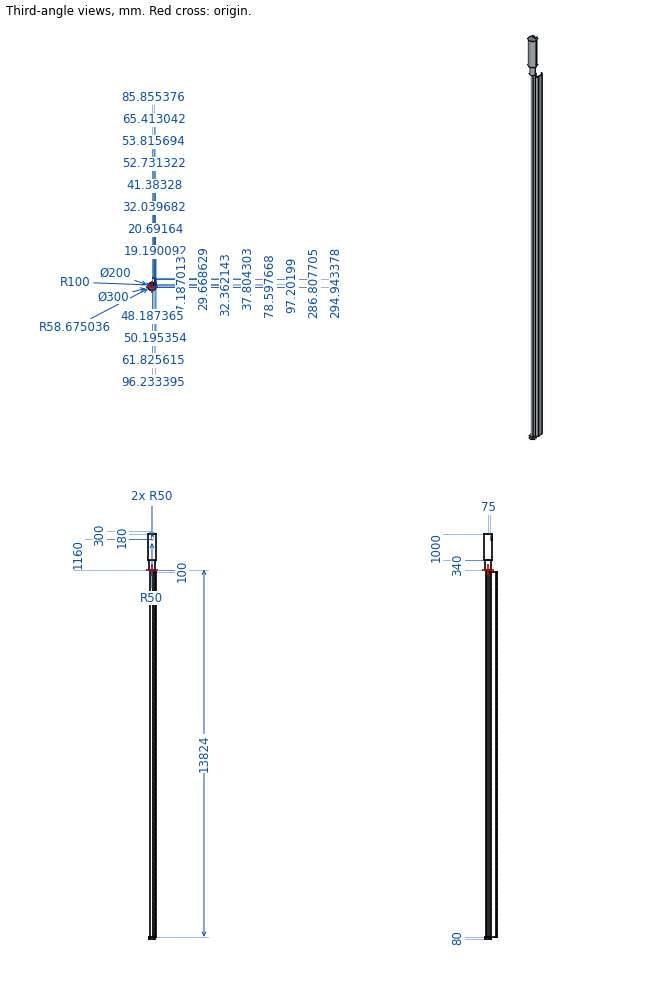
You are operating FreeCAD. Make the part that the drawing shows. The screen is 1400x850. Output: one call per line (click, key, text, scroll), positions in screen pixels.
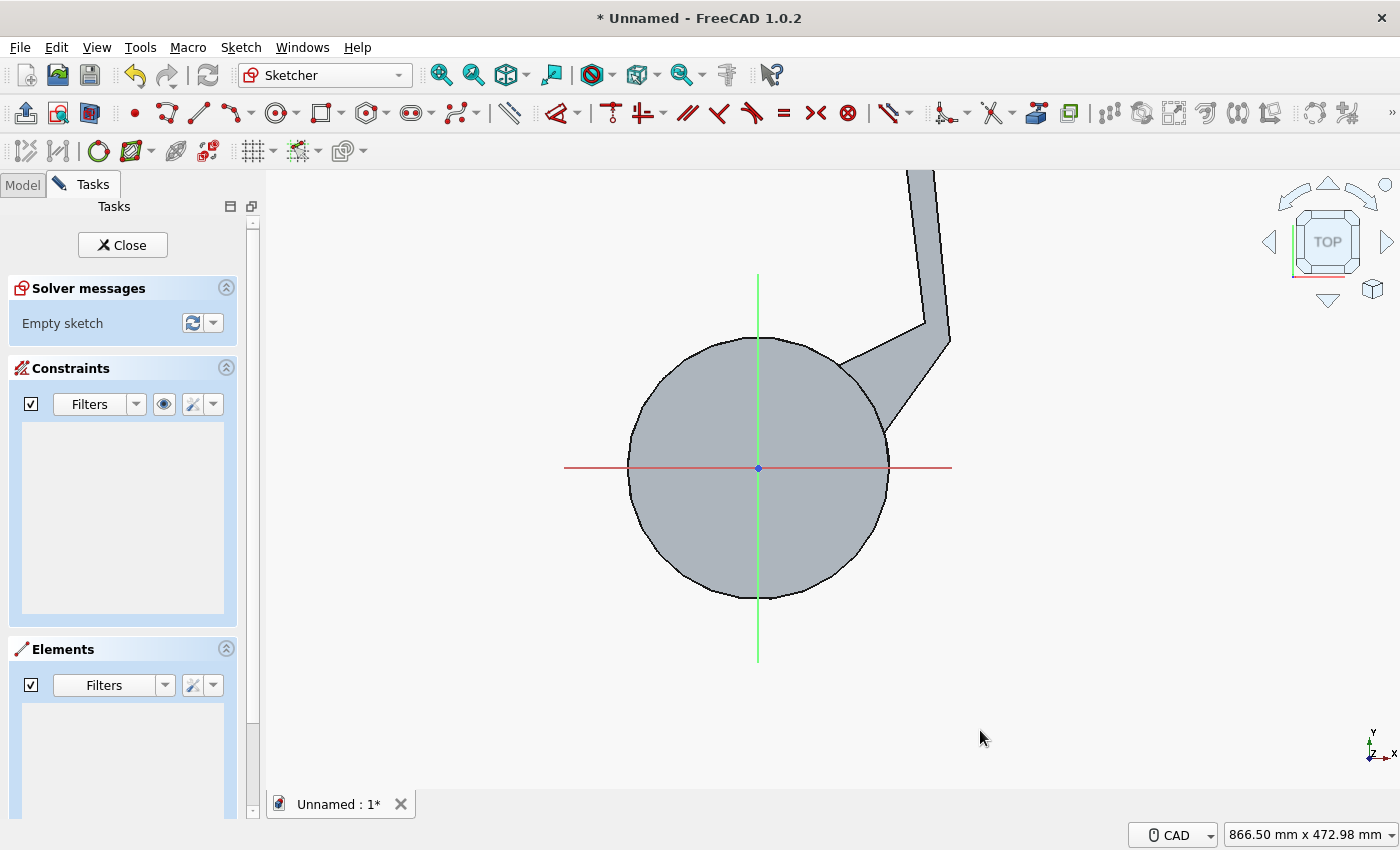
key(g)
key(c)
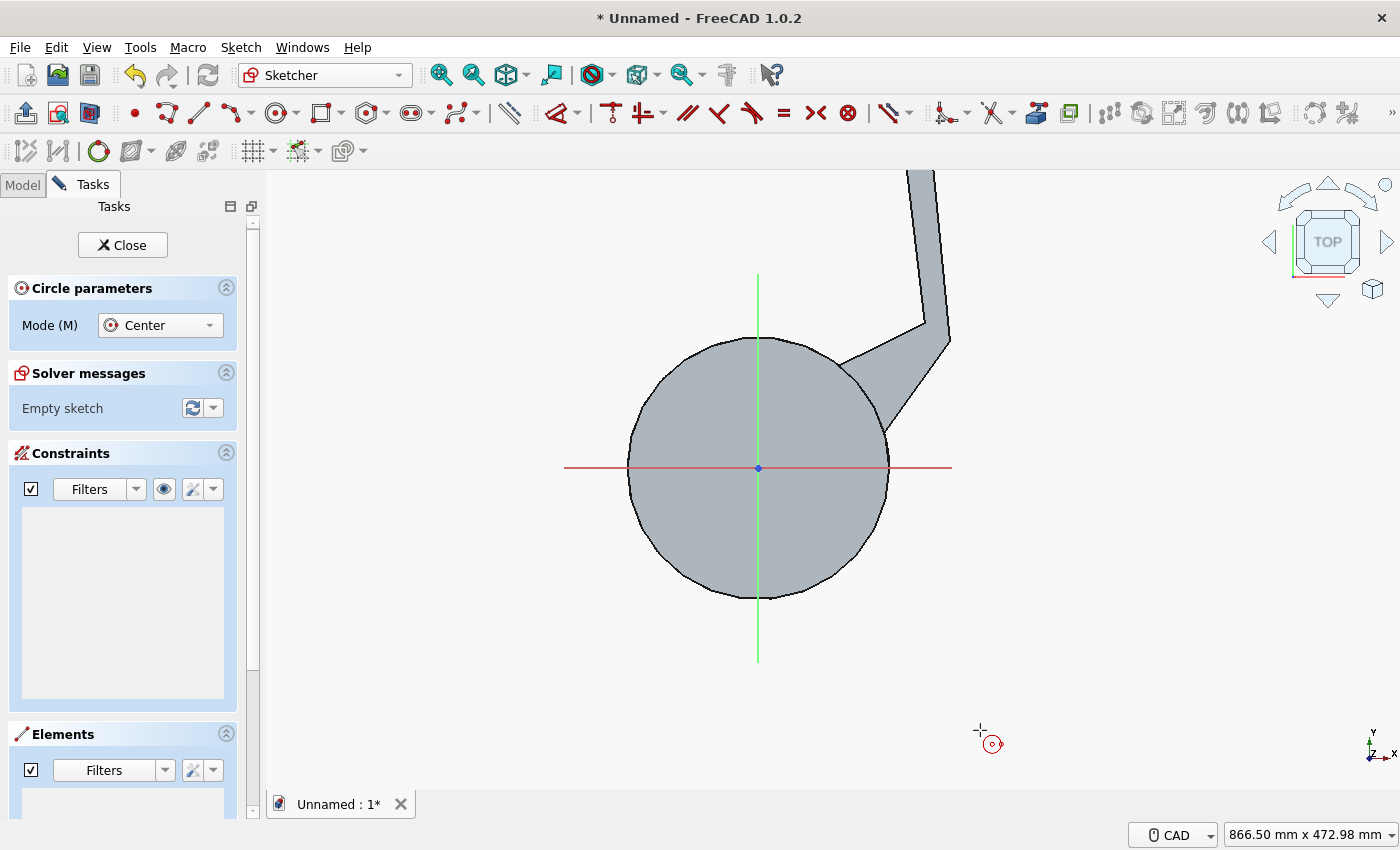
click(758, 468)
click(897, 330)
key(Escape)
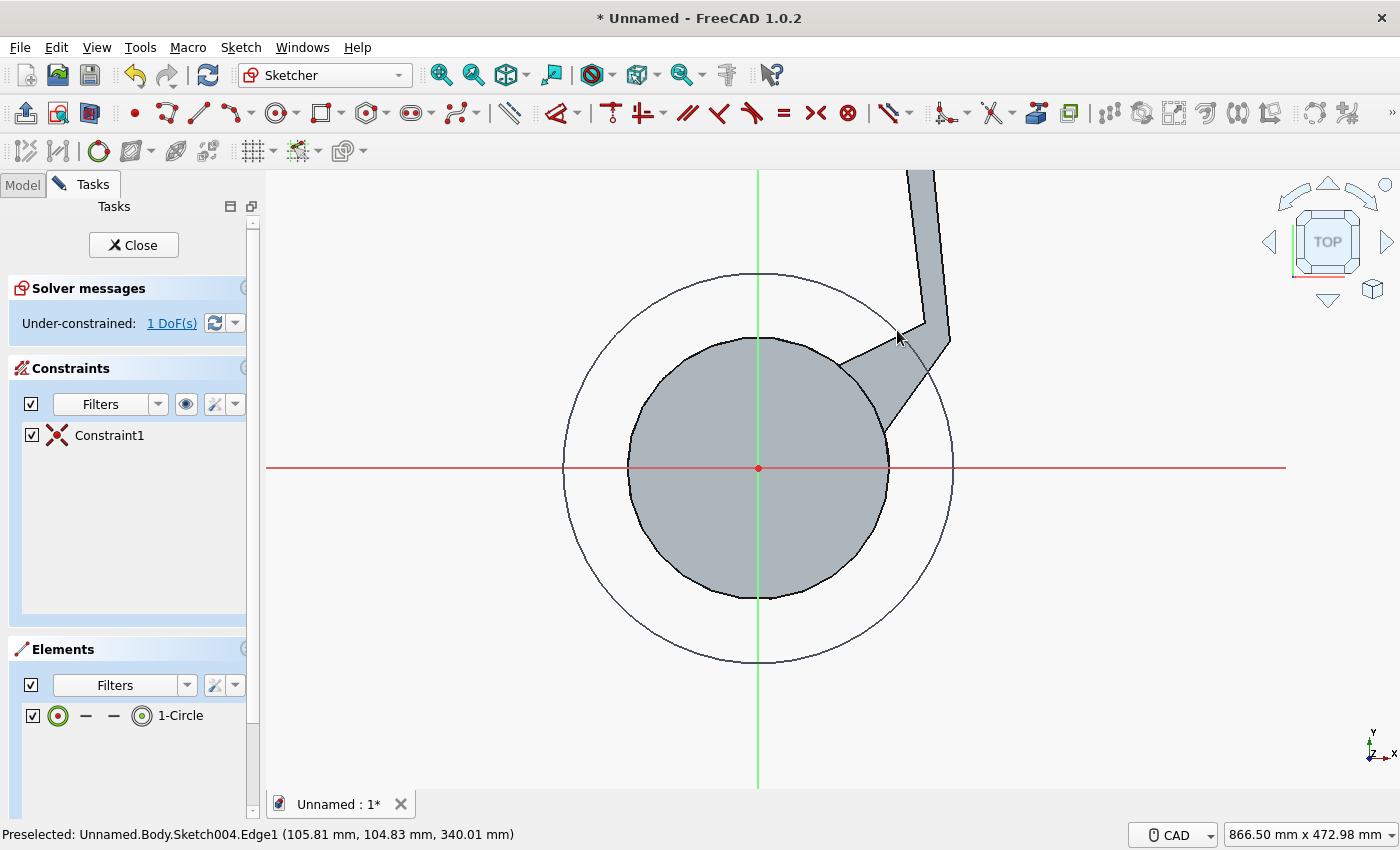
key(d)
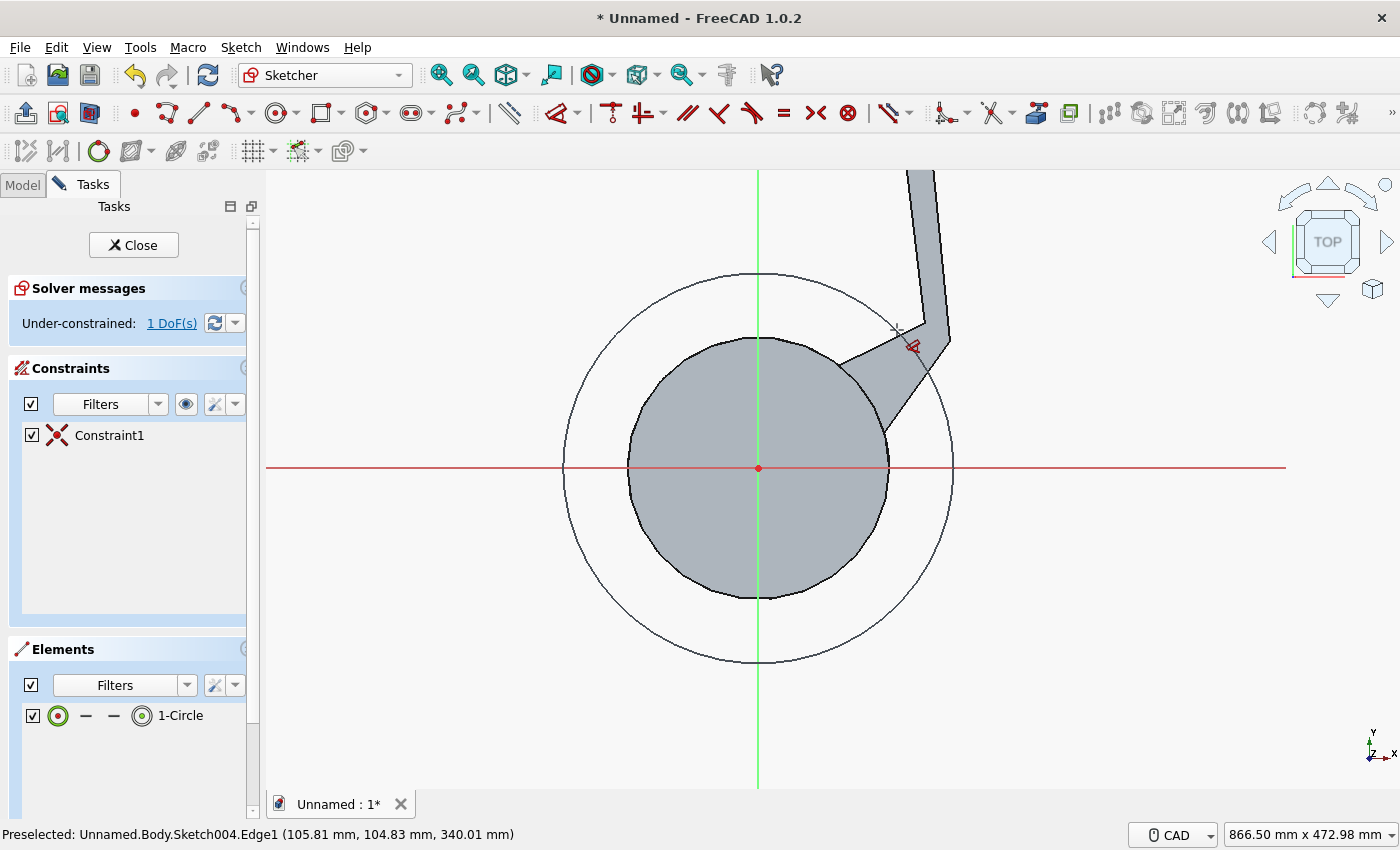
click(896, 330)
click(919, 307)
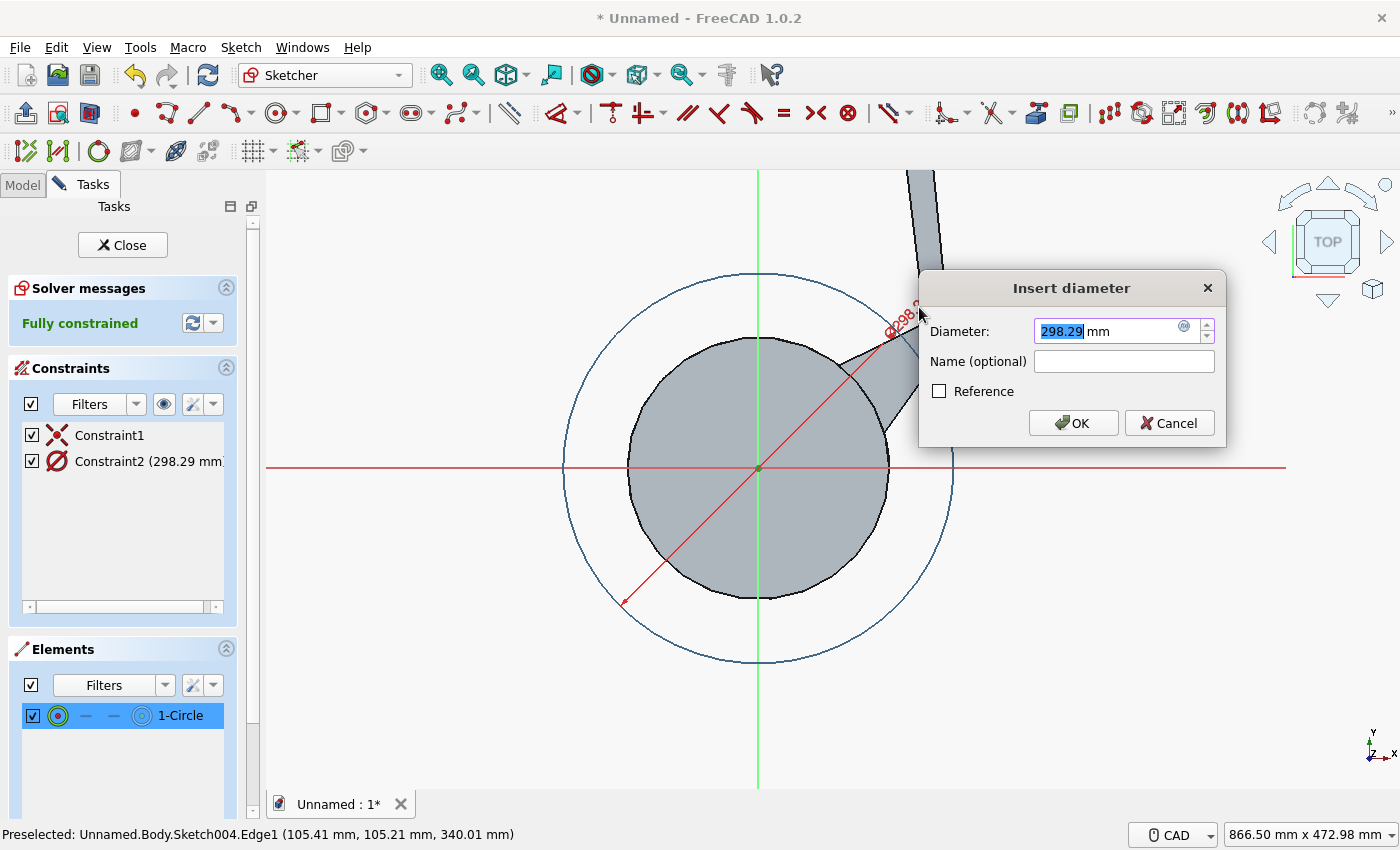
text(300)
key(Return)
key(Escape)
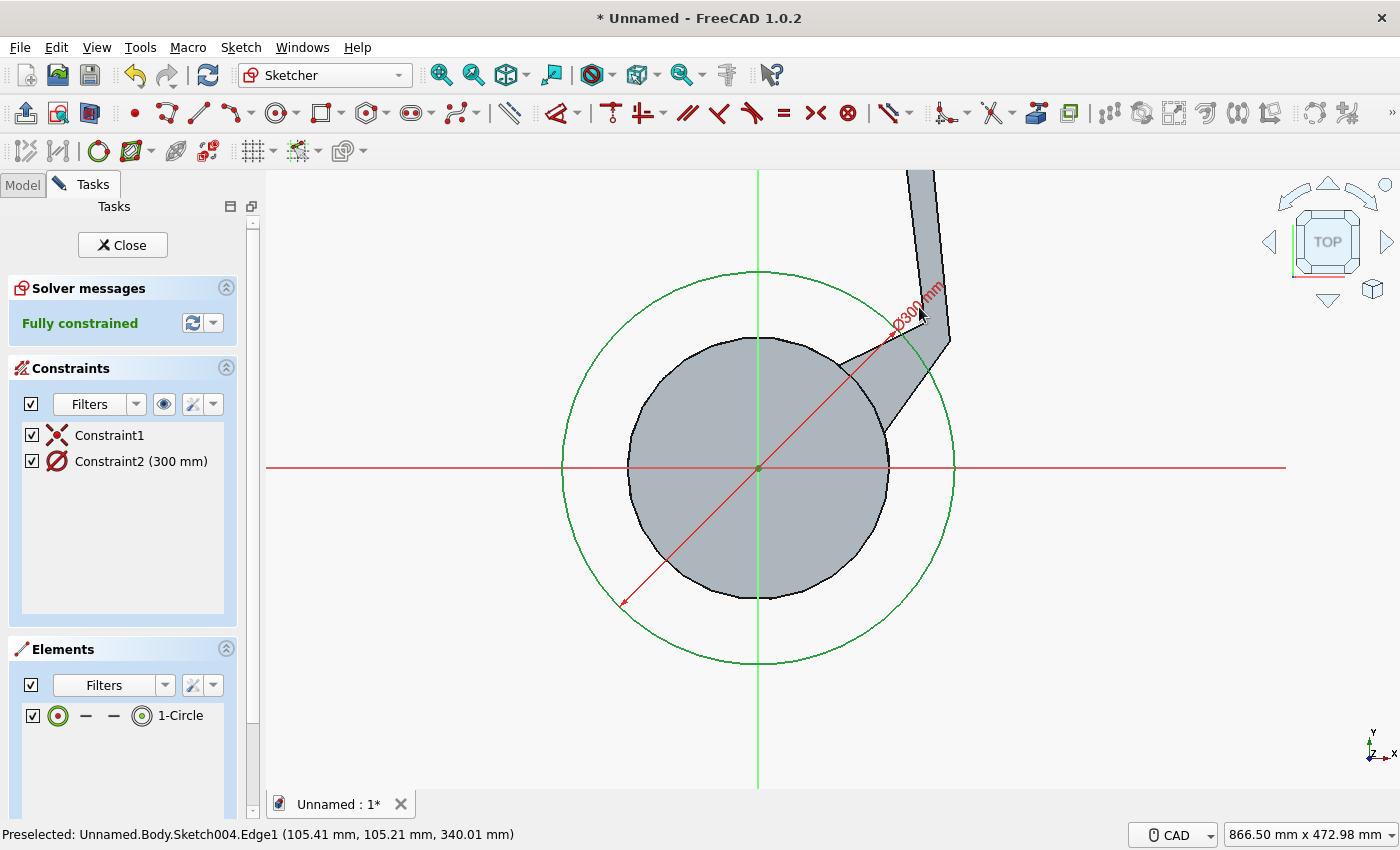
click(123, 245)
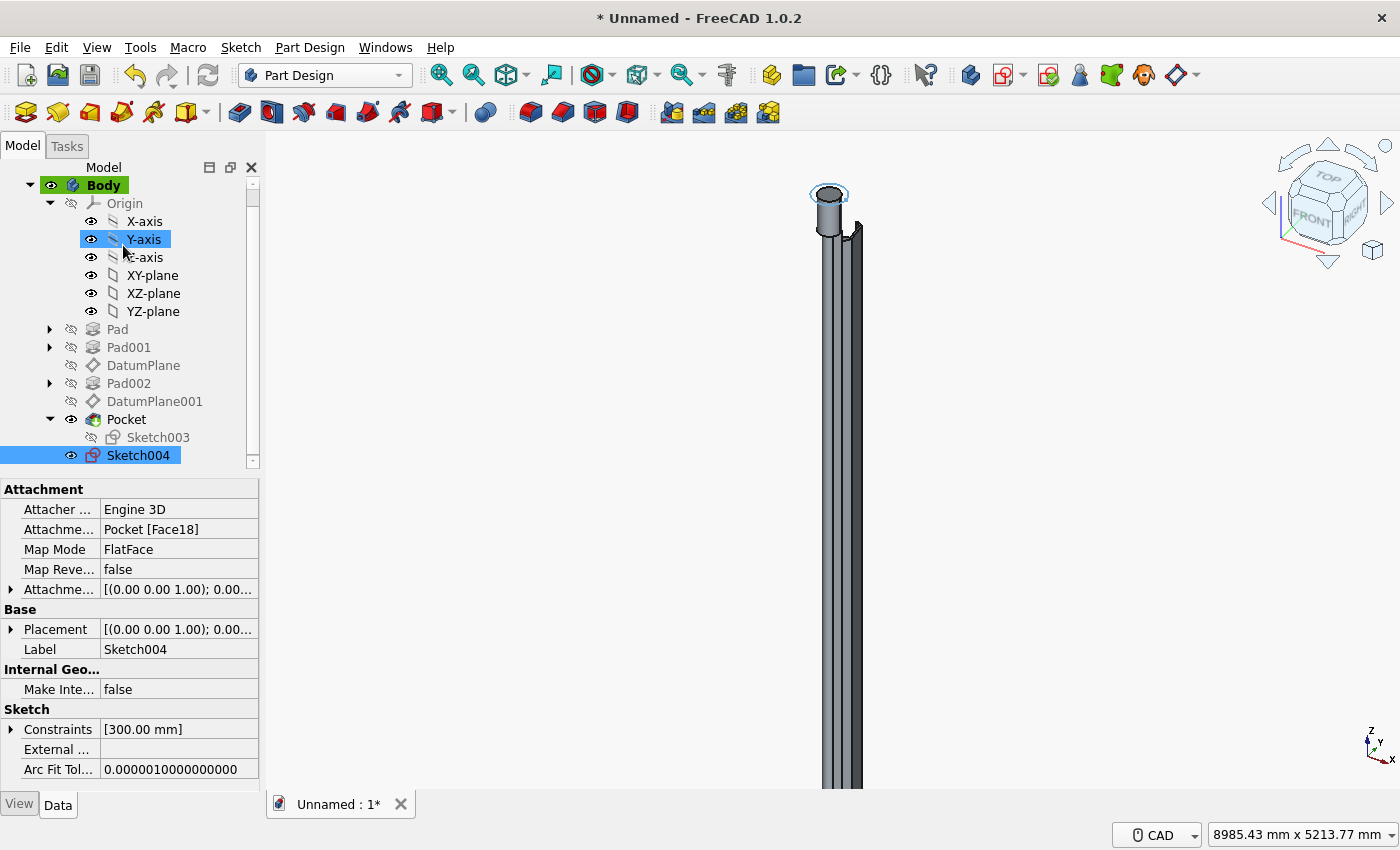
click(26, 112)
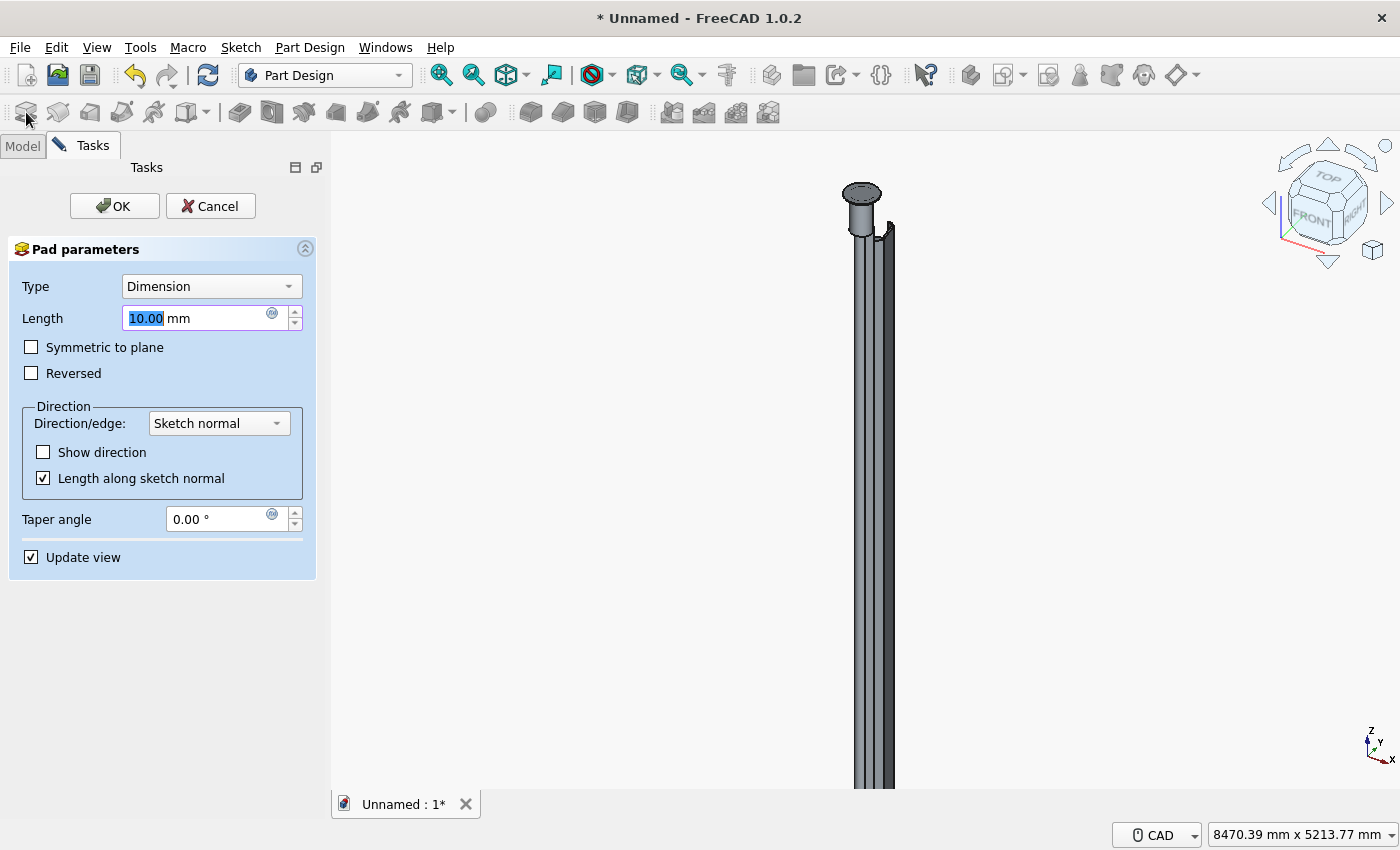
text(1000)
key(Tab)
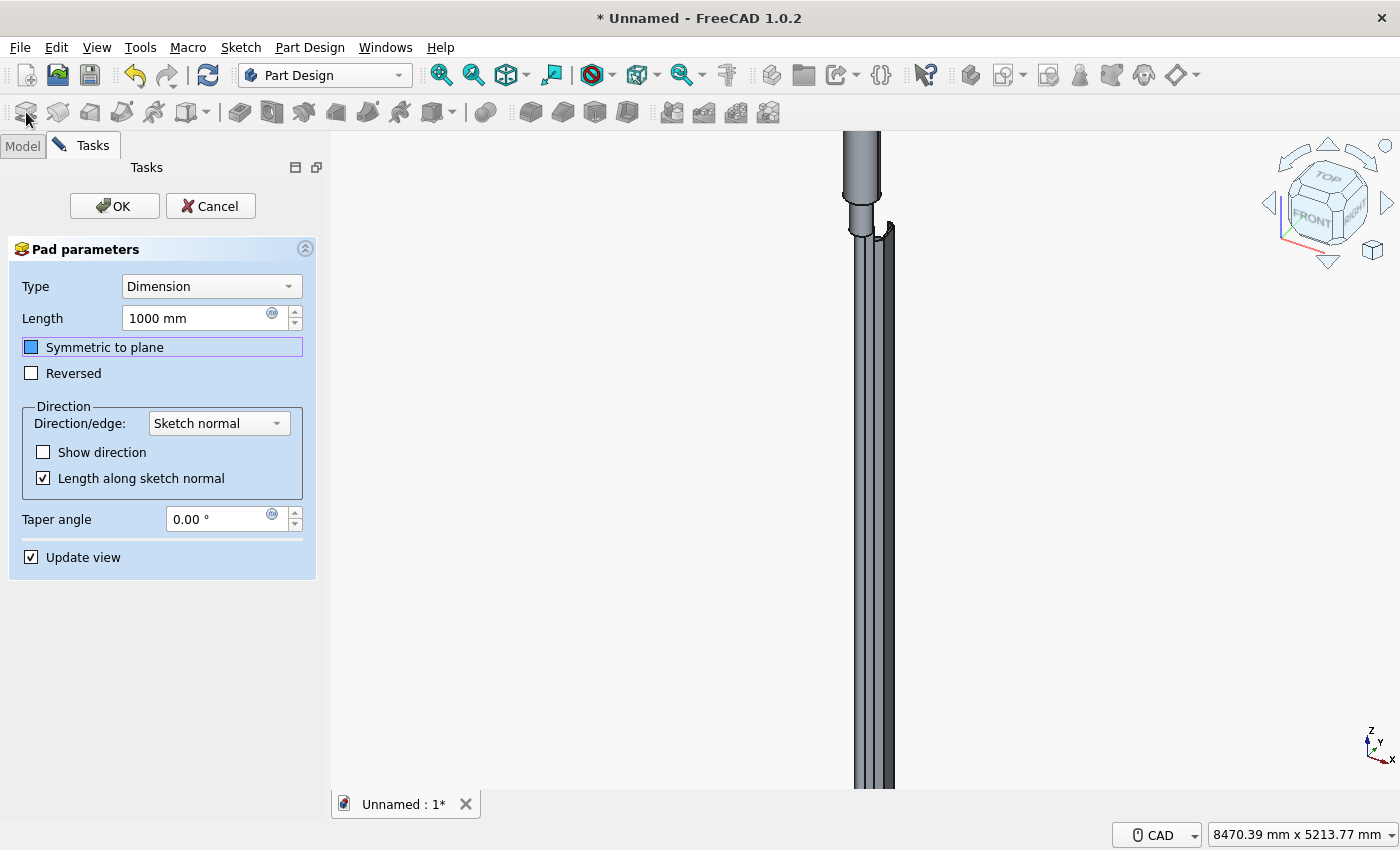
click(115, 206)